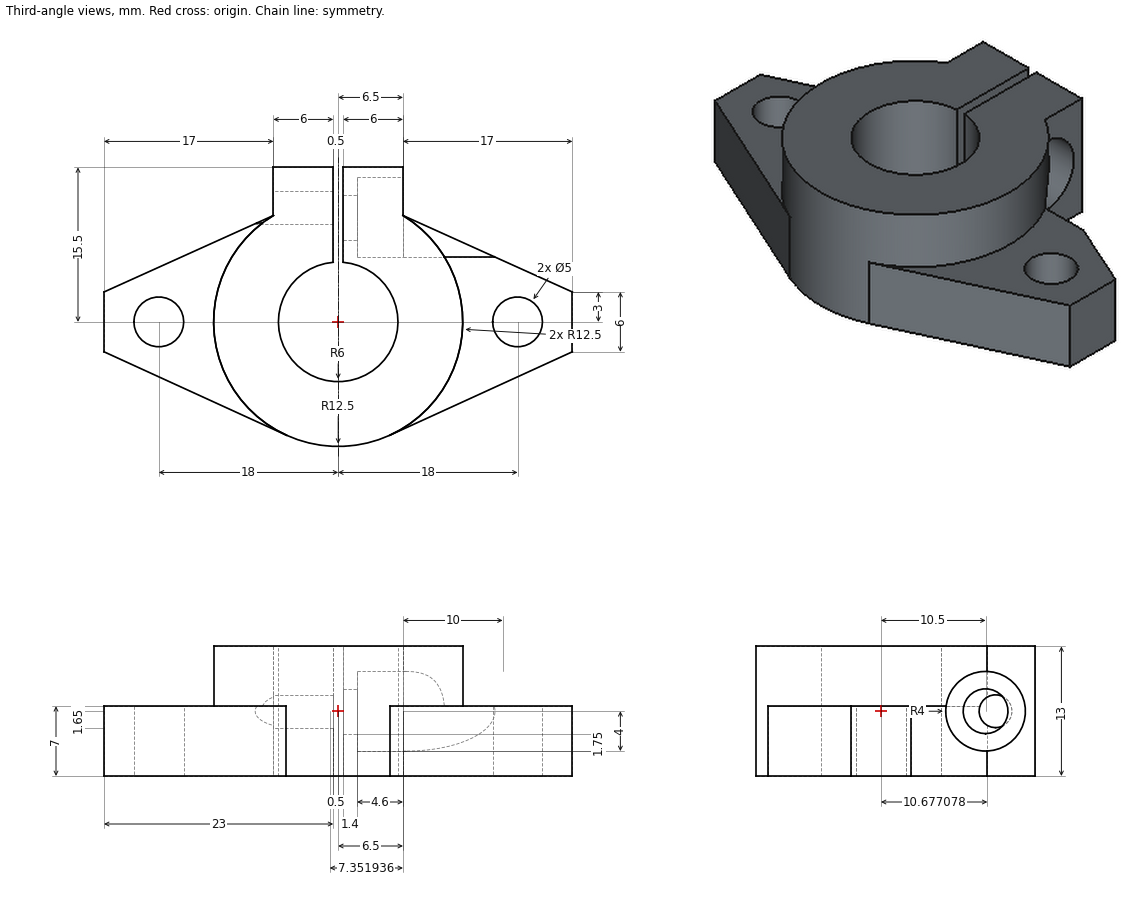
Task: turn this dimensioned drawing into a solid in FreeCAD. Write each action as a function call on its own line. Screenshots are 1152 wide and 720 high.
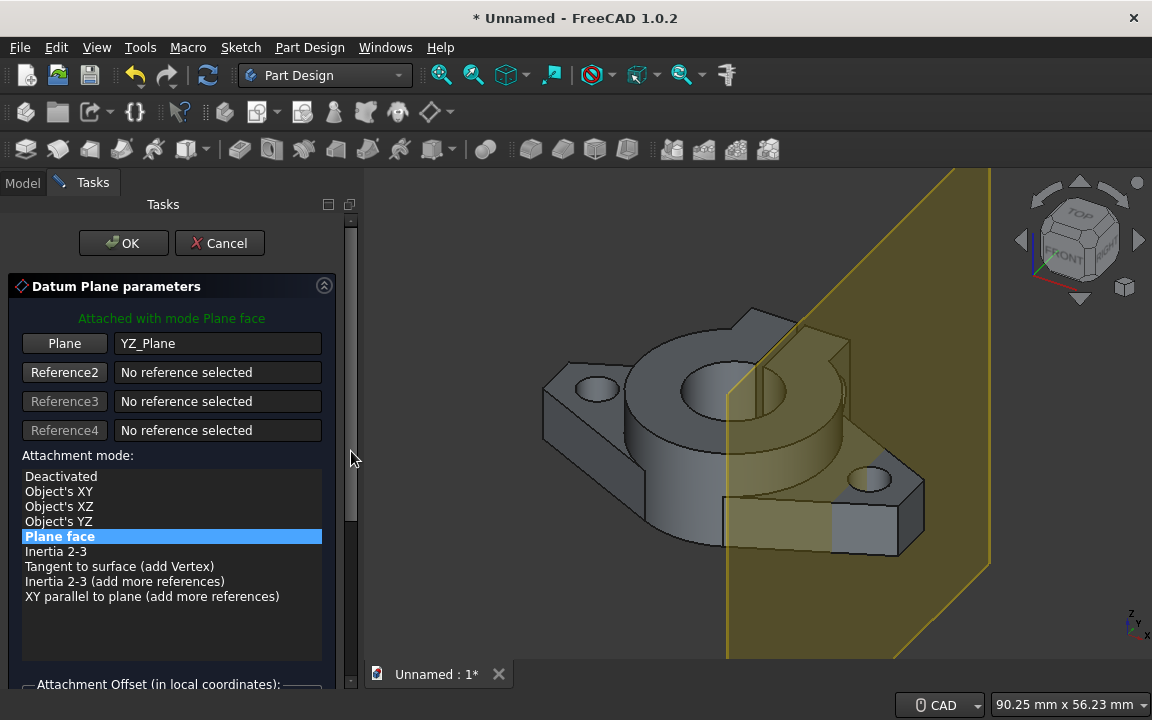
click(124, 243)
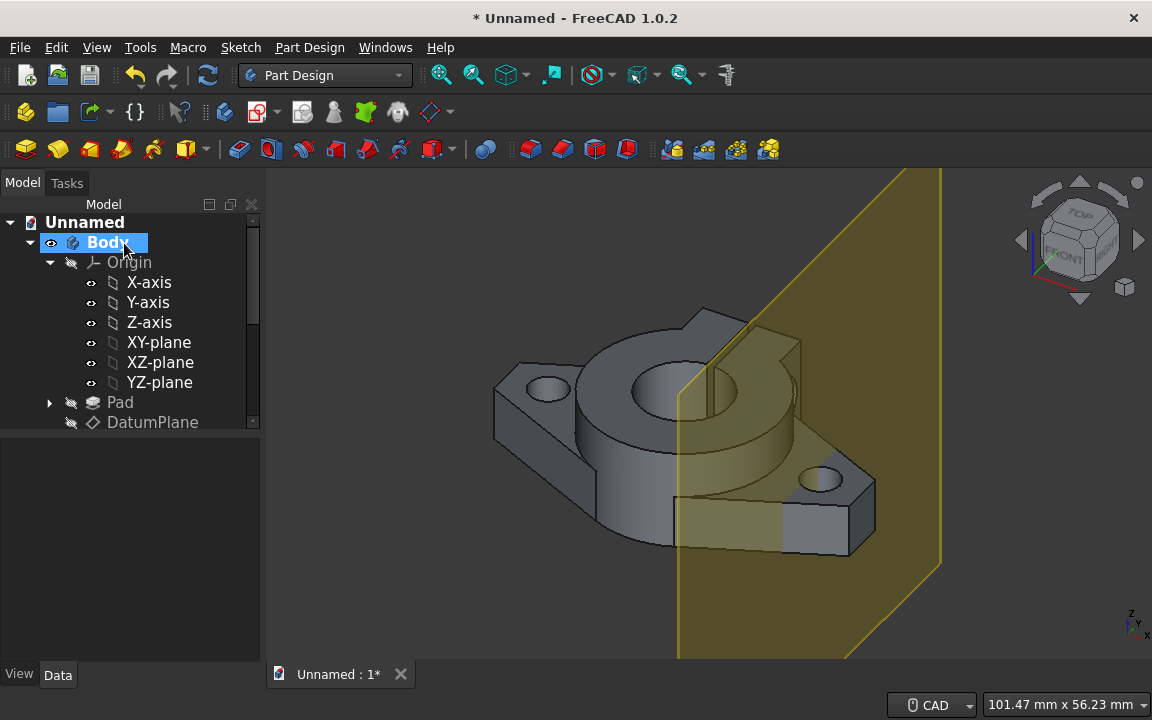
scroll(100, 318, down, 3)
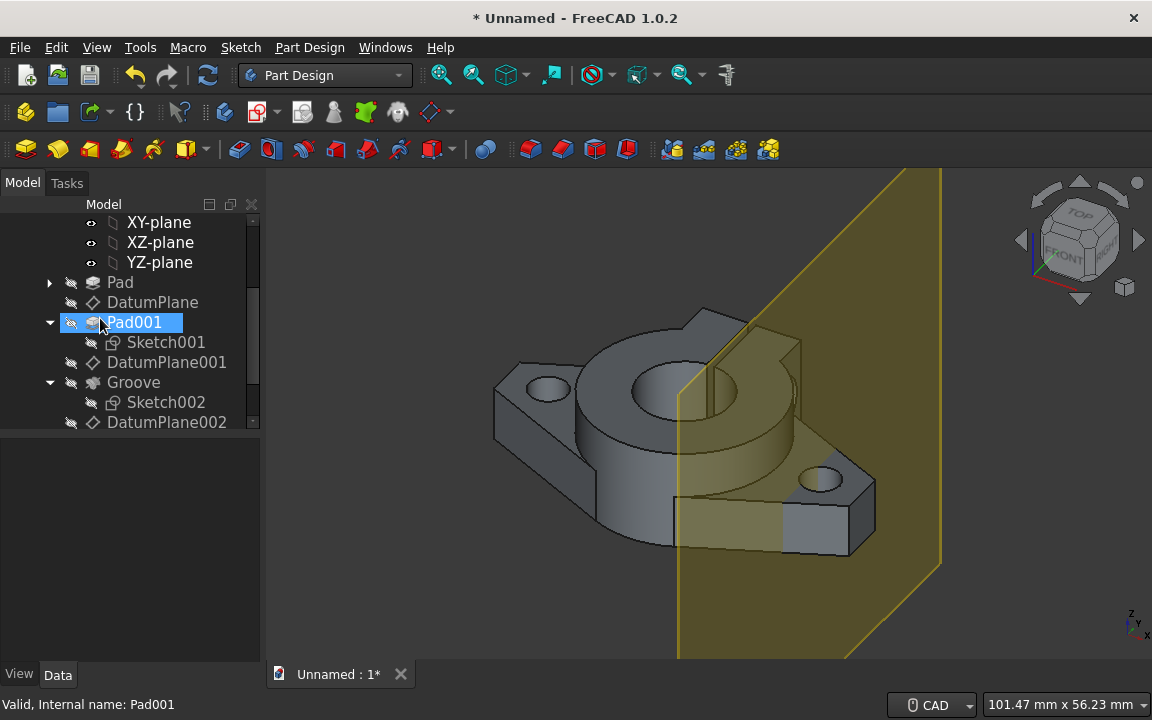
click(116, 403)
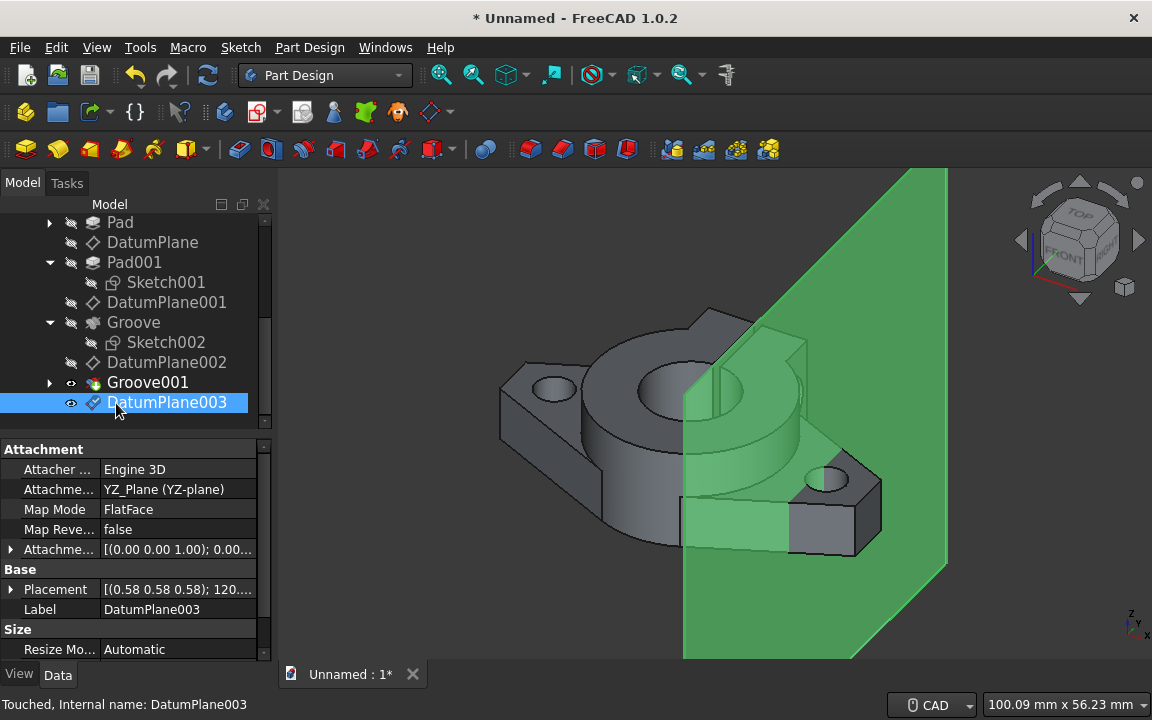
click(258, 112)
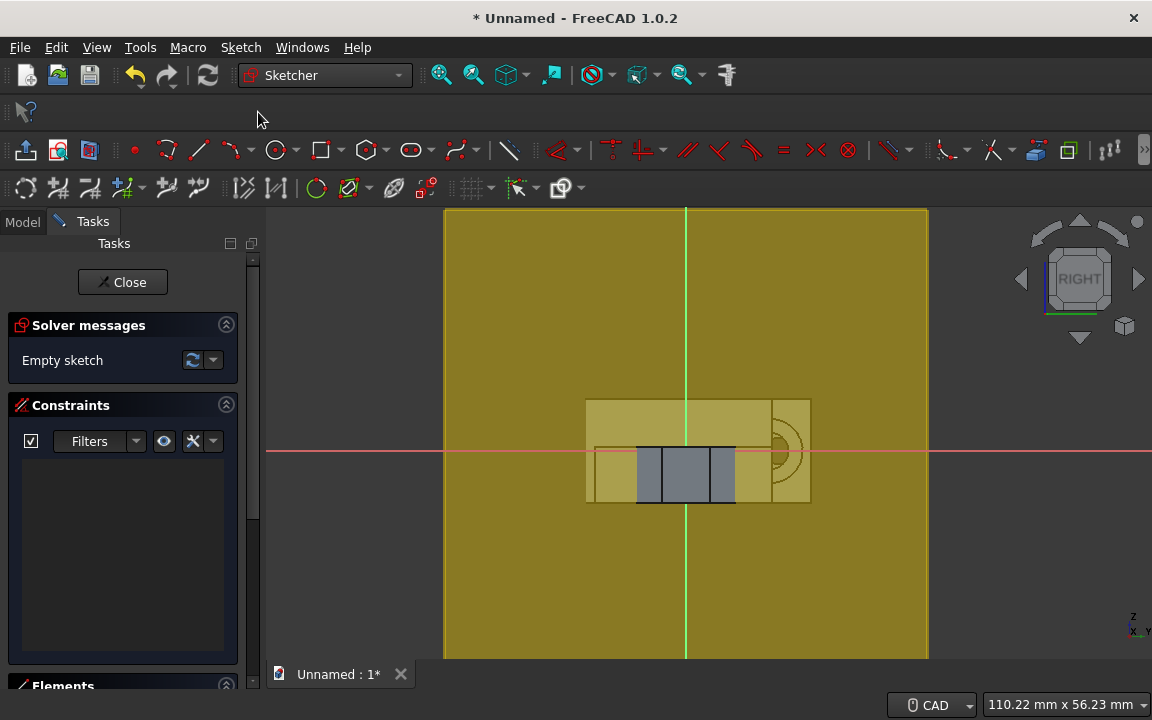
click(90, 150)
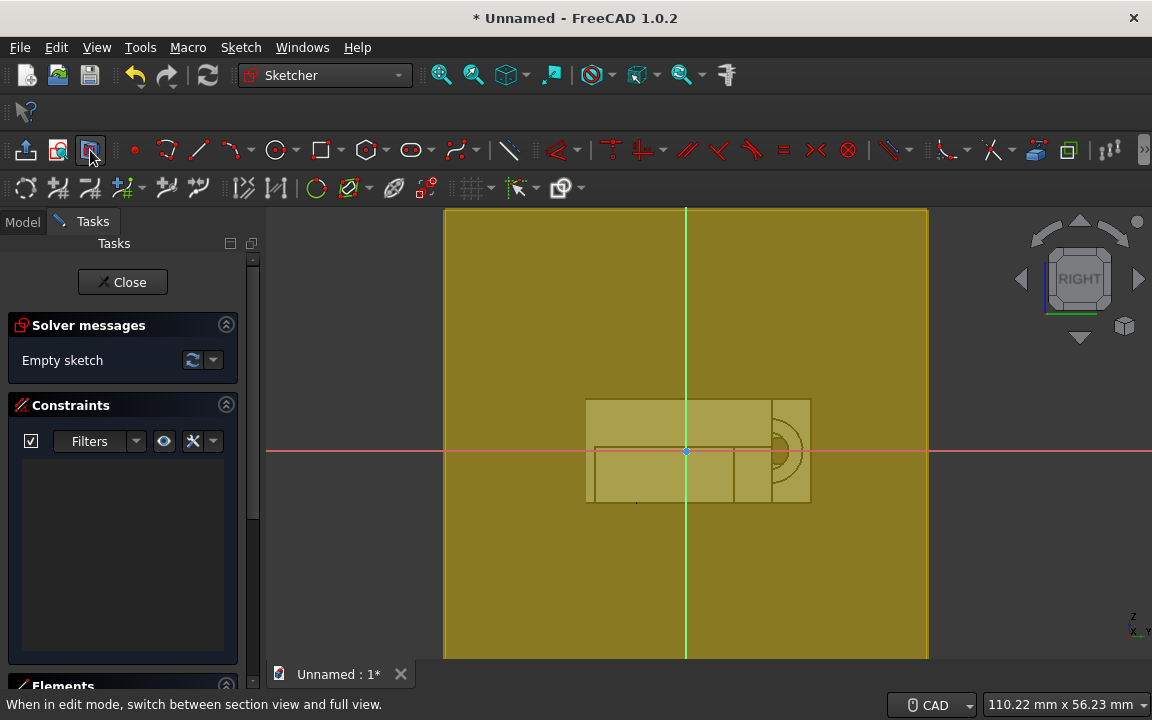
scroll(758, 457, up, 7)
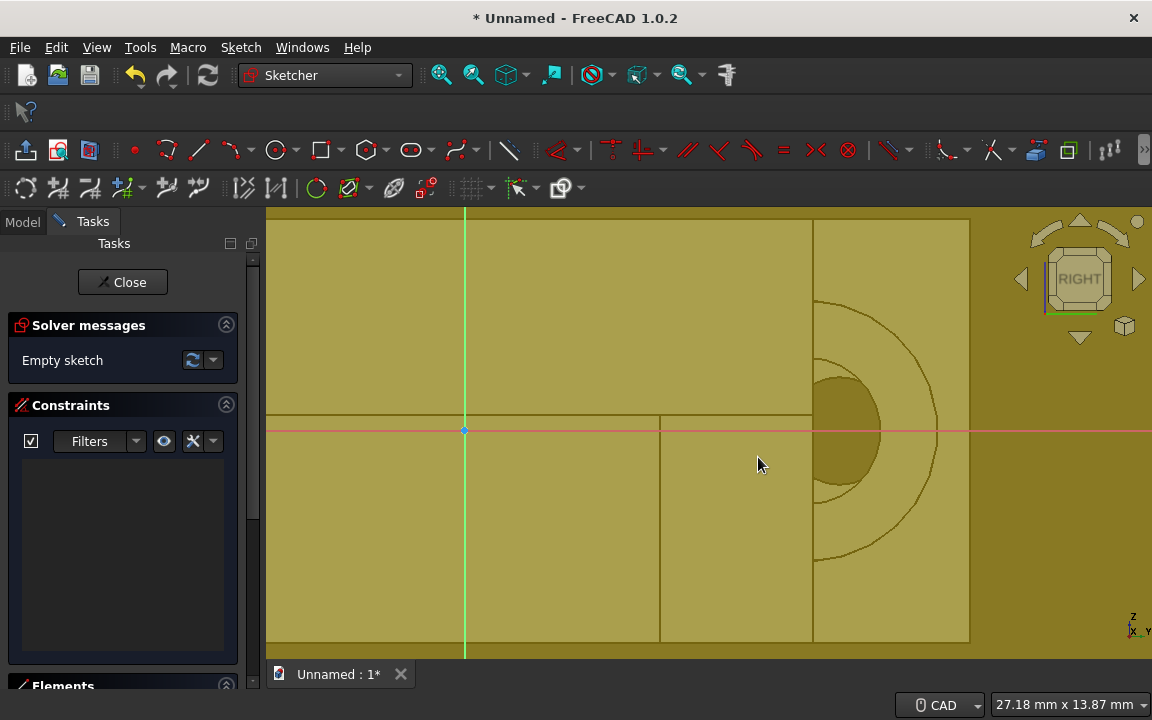
click(200, 150)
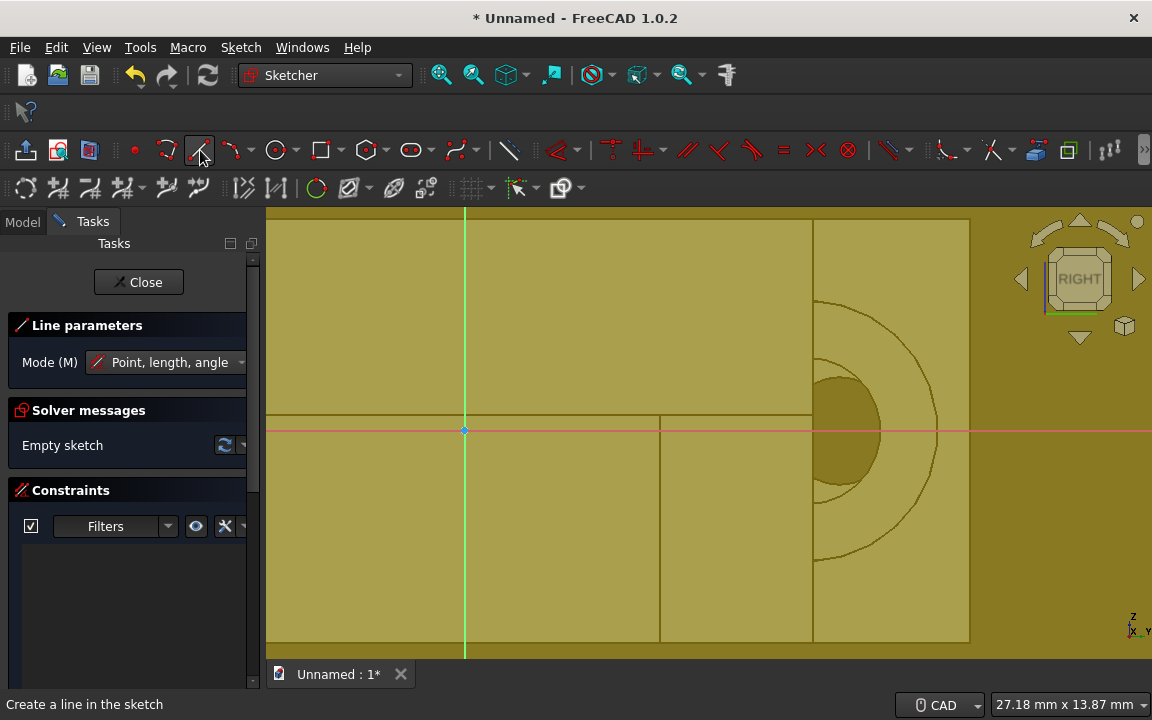
click(813, 561)
click(813, 301)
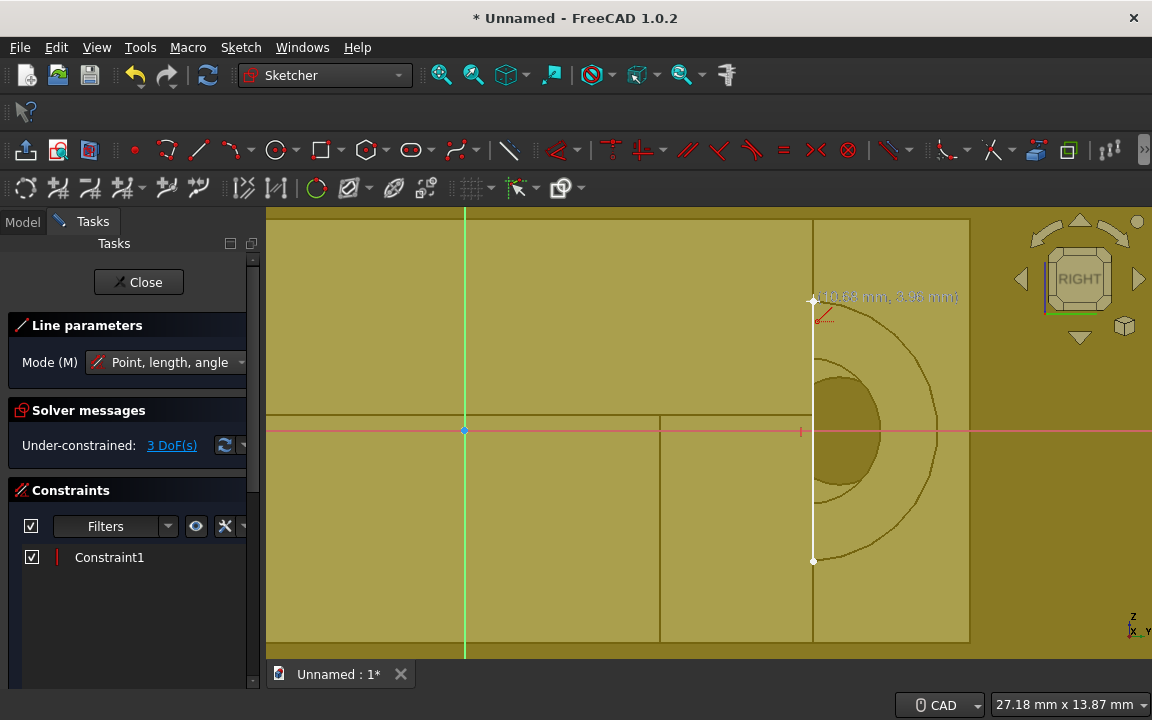
click(232, 150)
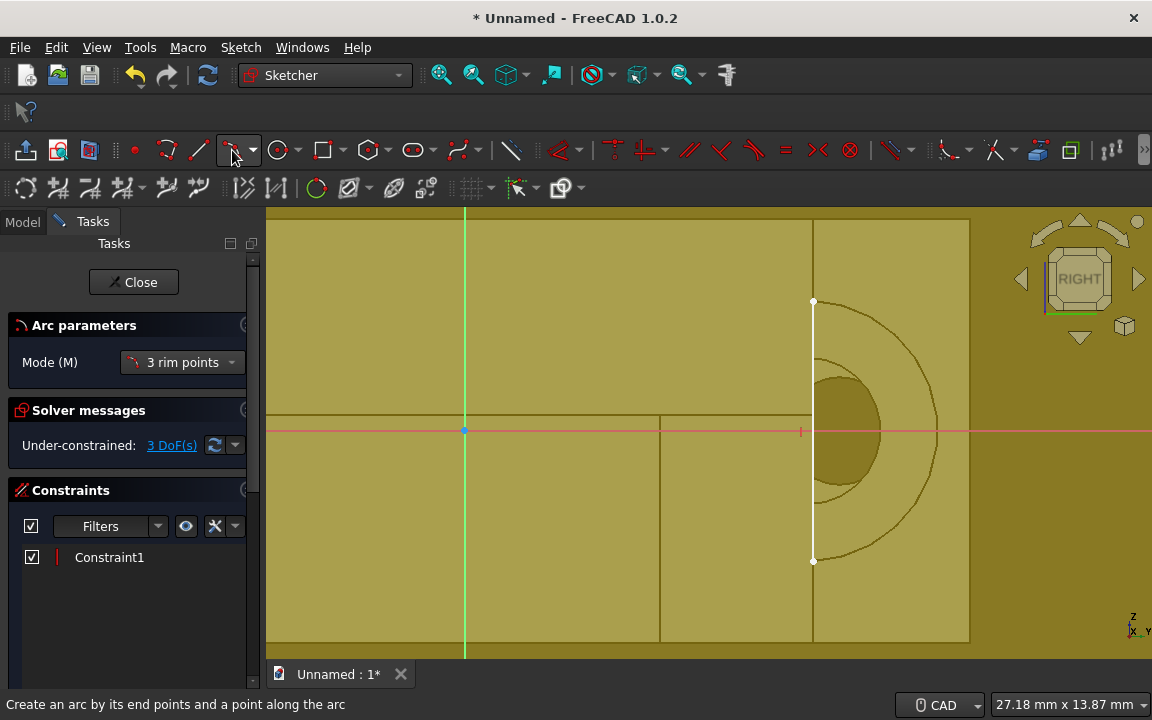
click(813, 302)
click(813, 562)
click(684, 390)
key(Escape)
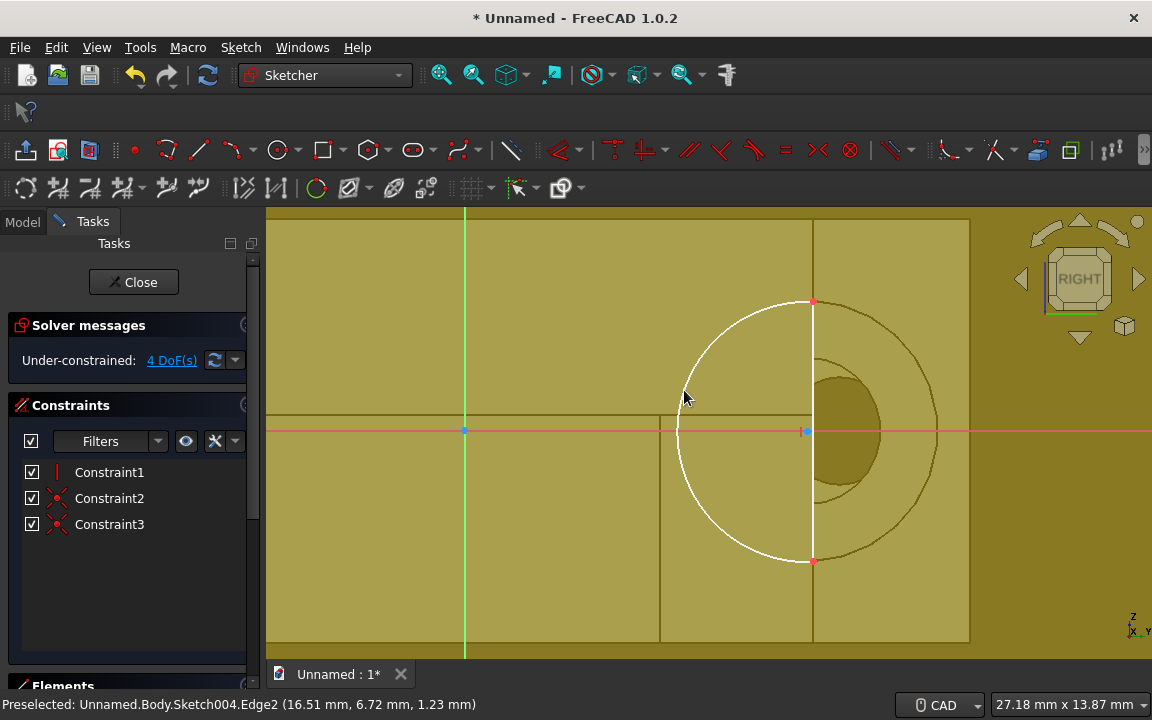
click(807, 432)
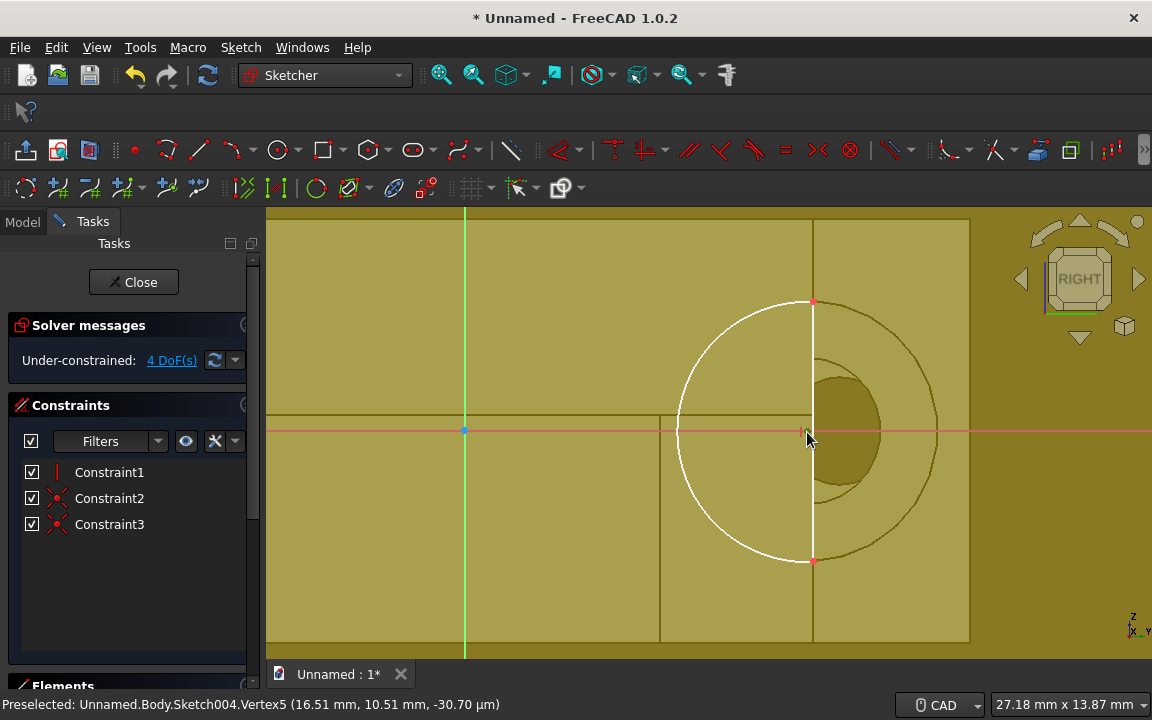
click(344, 431)